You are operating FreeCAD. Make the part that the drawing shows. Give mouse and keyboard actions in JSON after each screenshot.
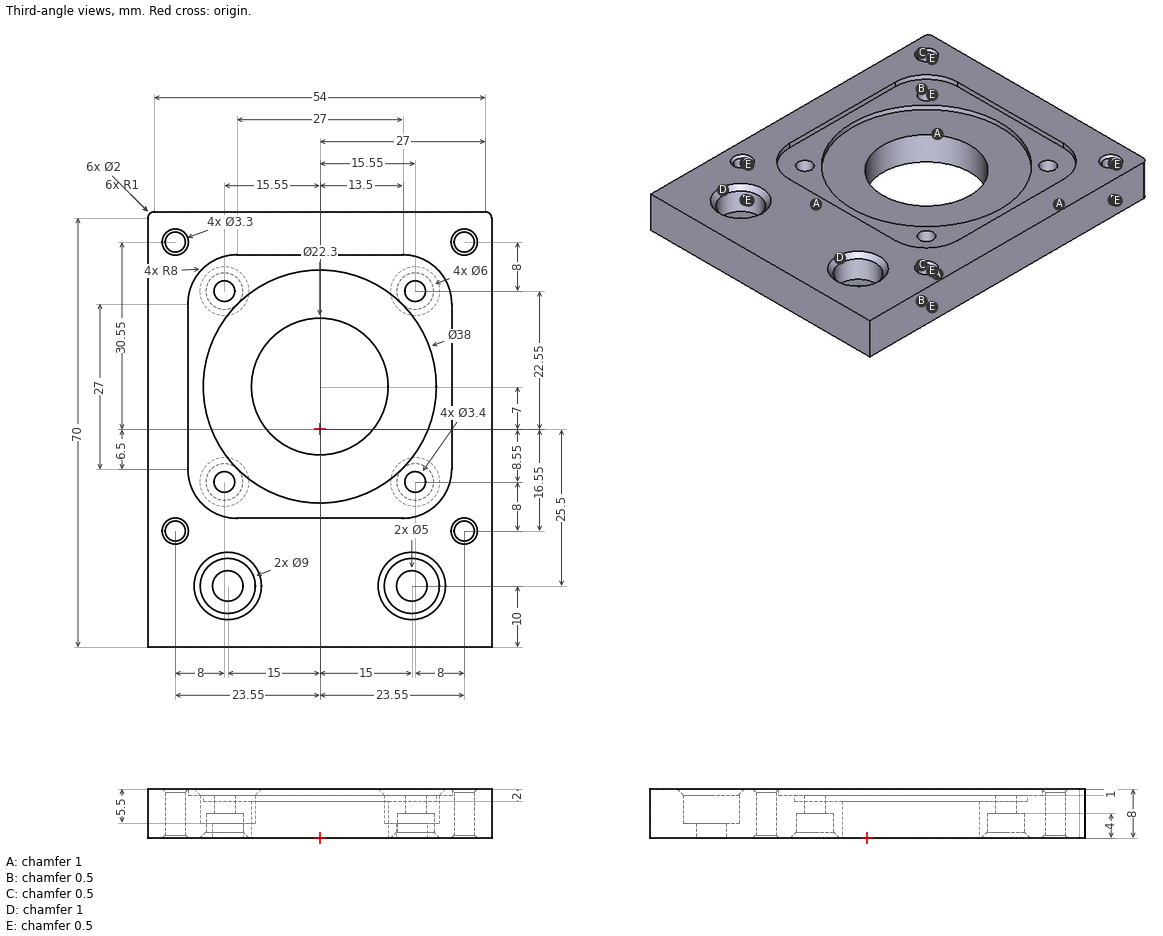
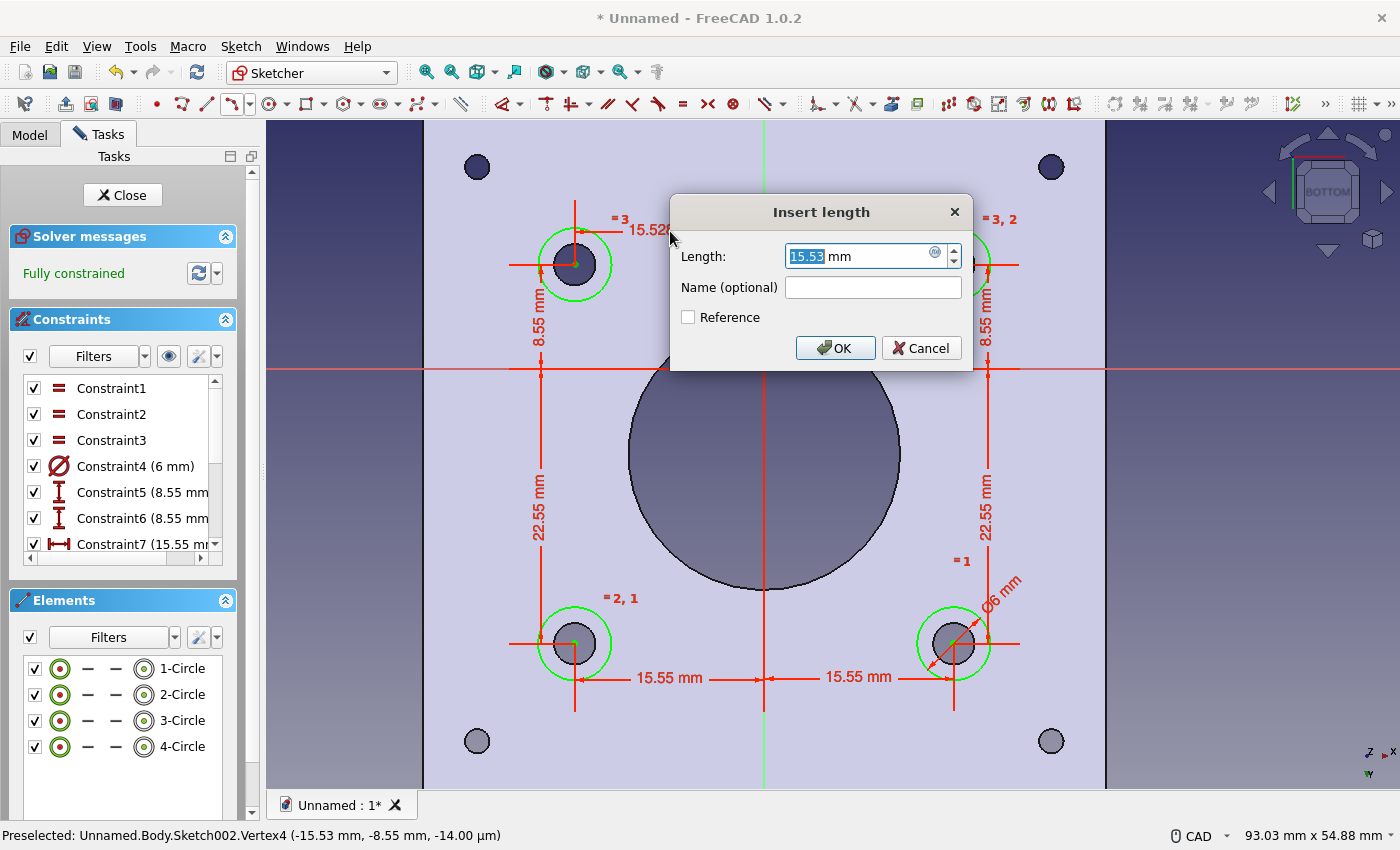
{"action": "type", "text": "15.55"}
{"action": "key", "text": "Return"}
{"action": "key", "text": "Escape"}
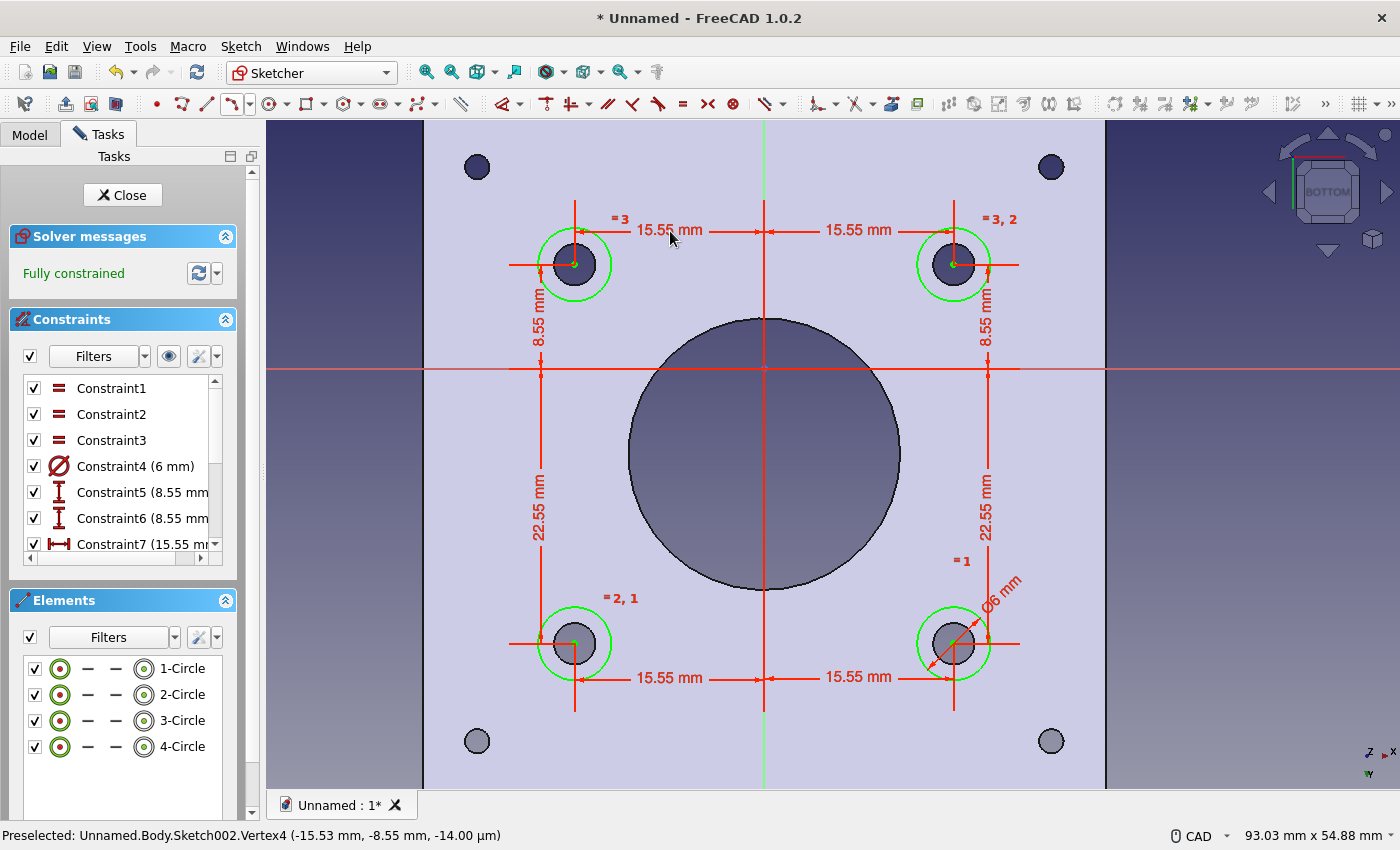
{"action": "left_click", "coordinate": [123, 195]}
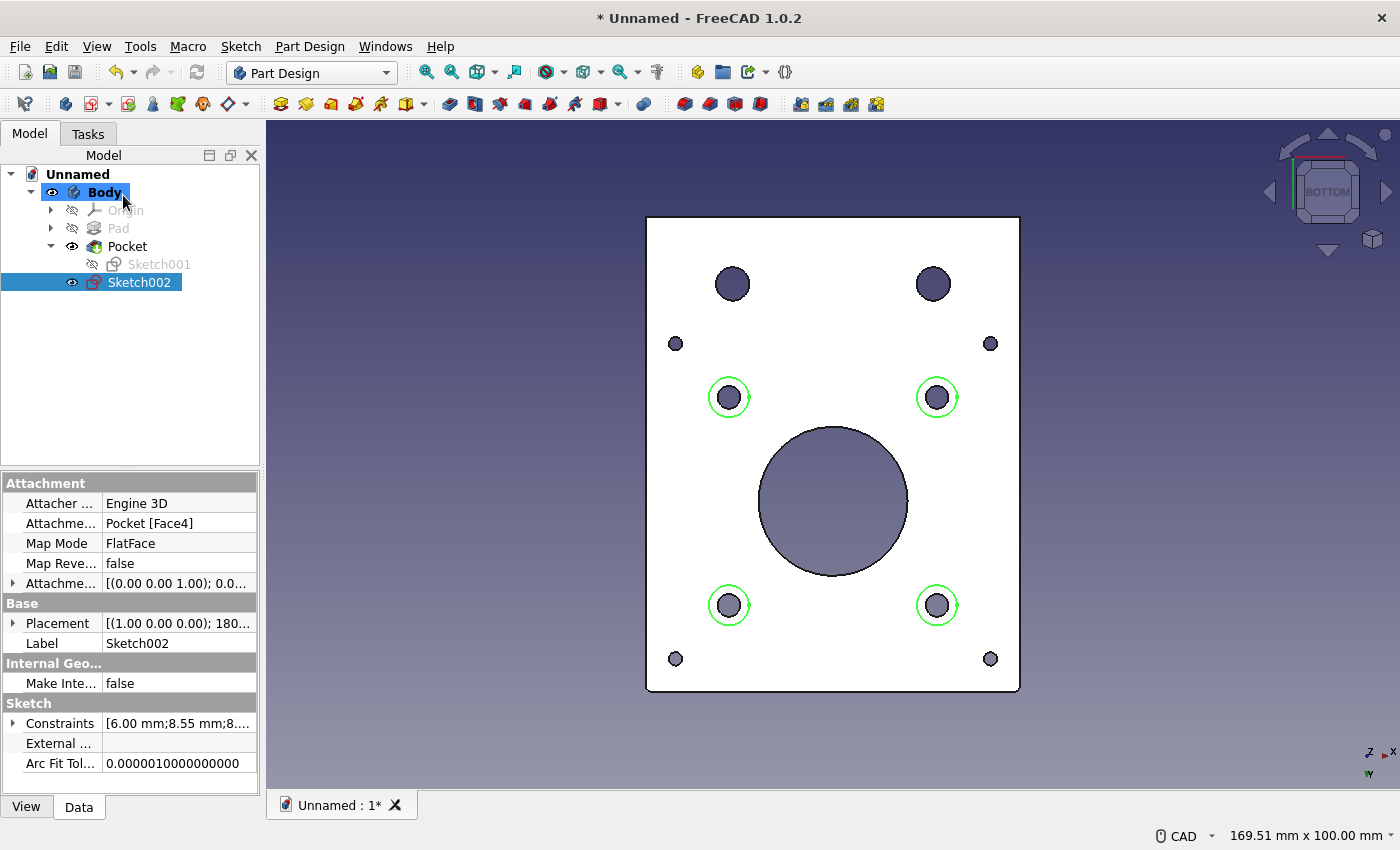
{"action": "left_click", "coordinate": [450, 104]}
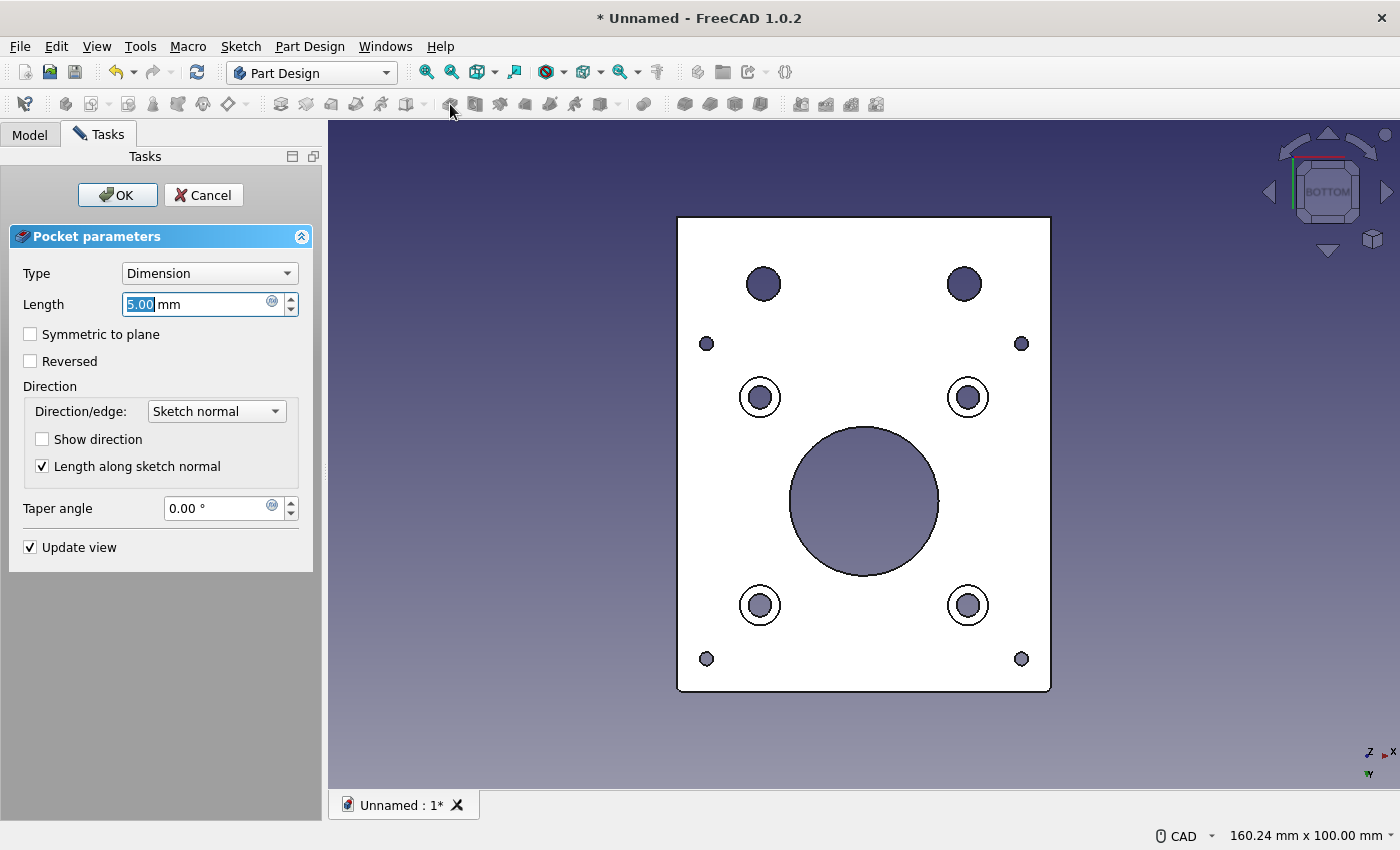
{"action": "type", "text": "4"}
{"action": "key", "text": "Tab"}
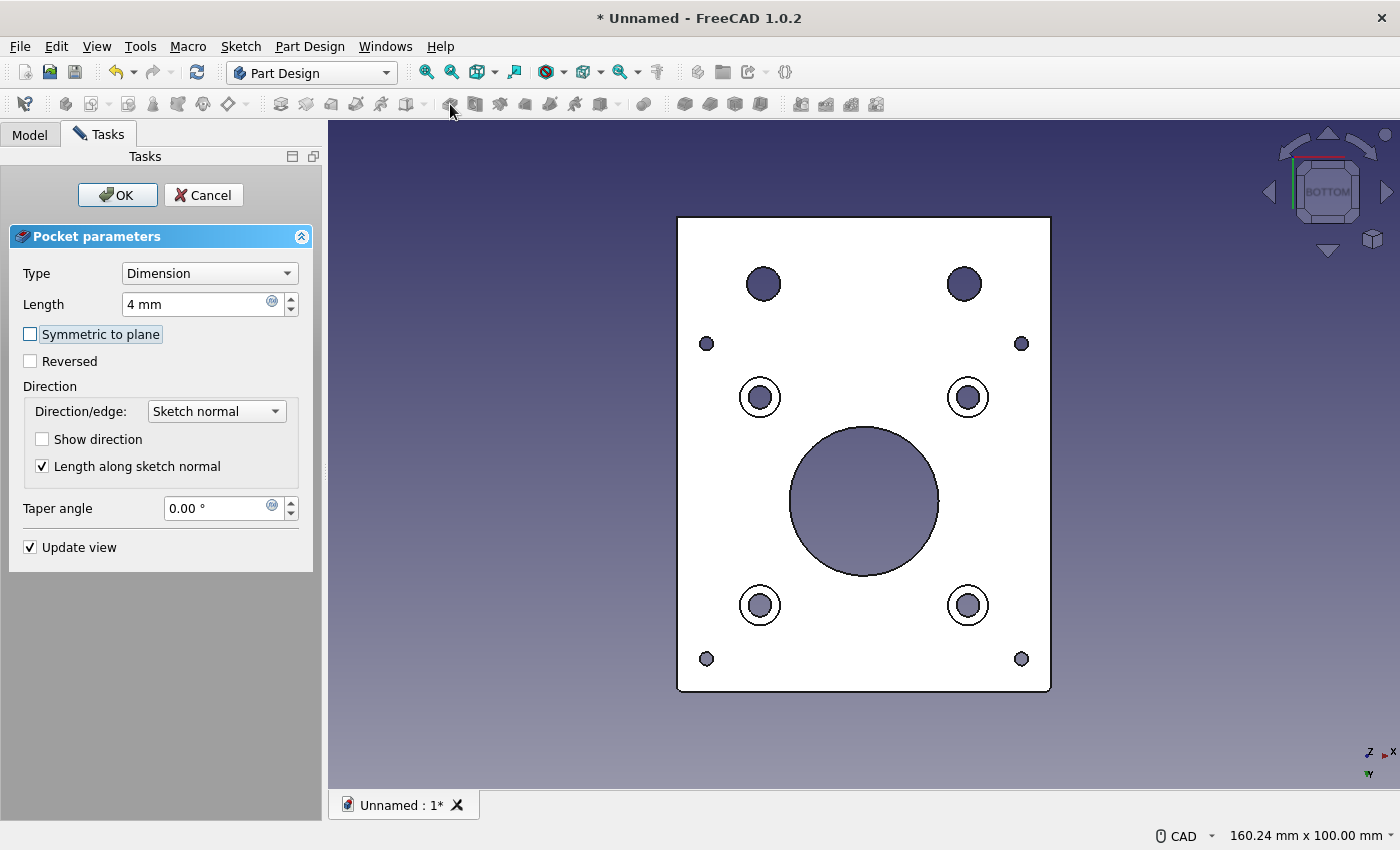
{"action": "left_click", "coordinate": [118, 195]}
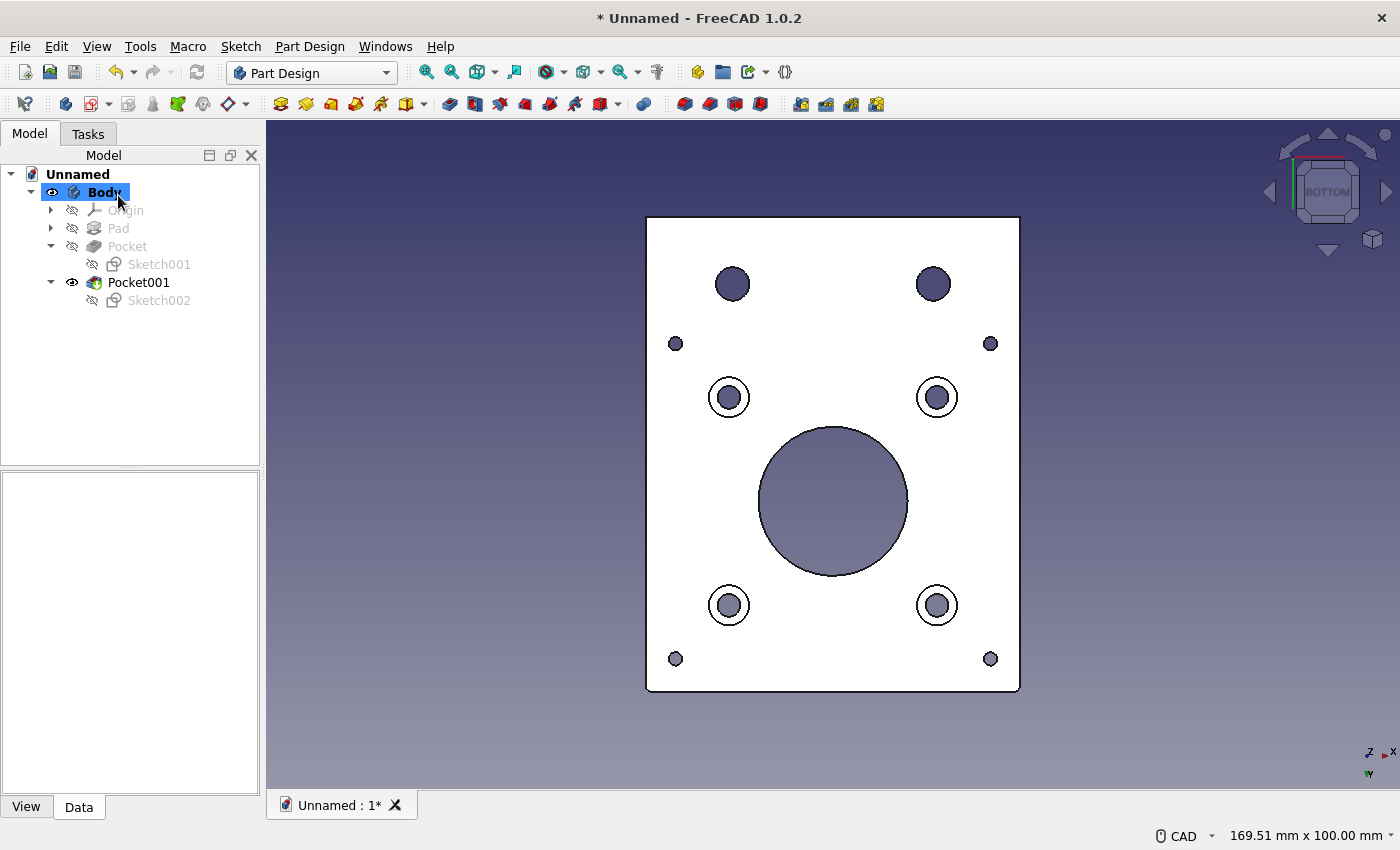
{"action": "left_click", "coordinate": [917, 604]}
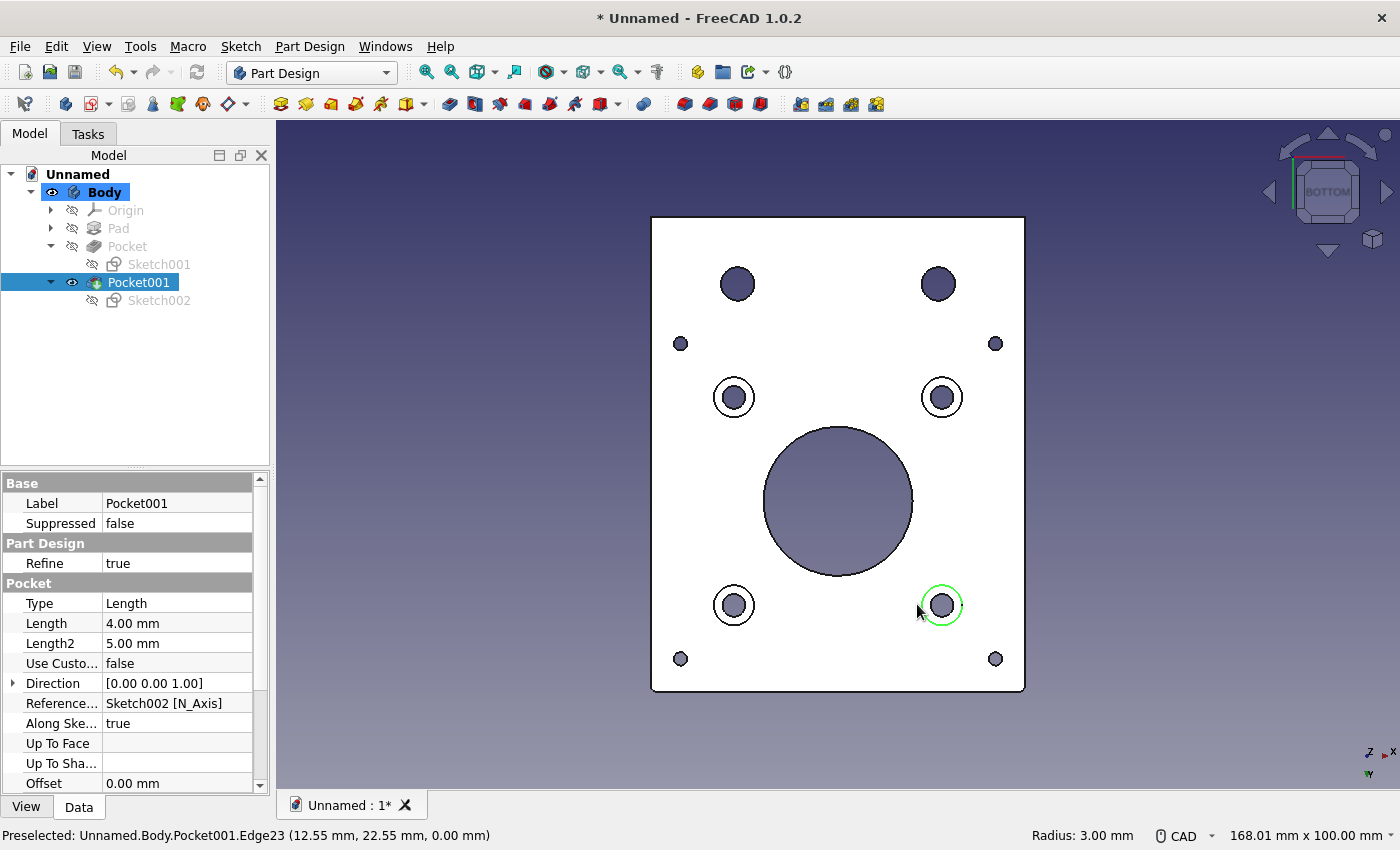
{"action": "left_click", "coordinate": [714, 604], "text": "ctrl"}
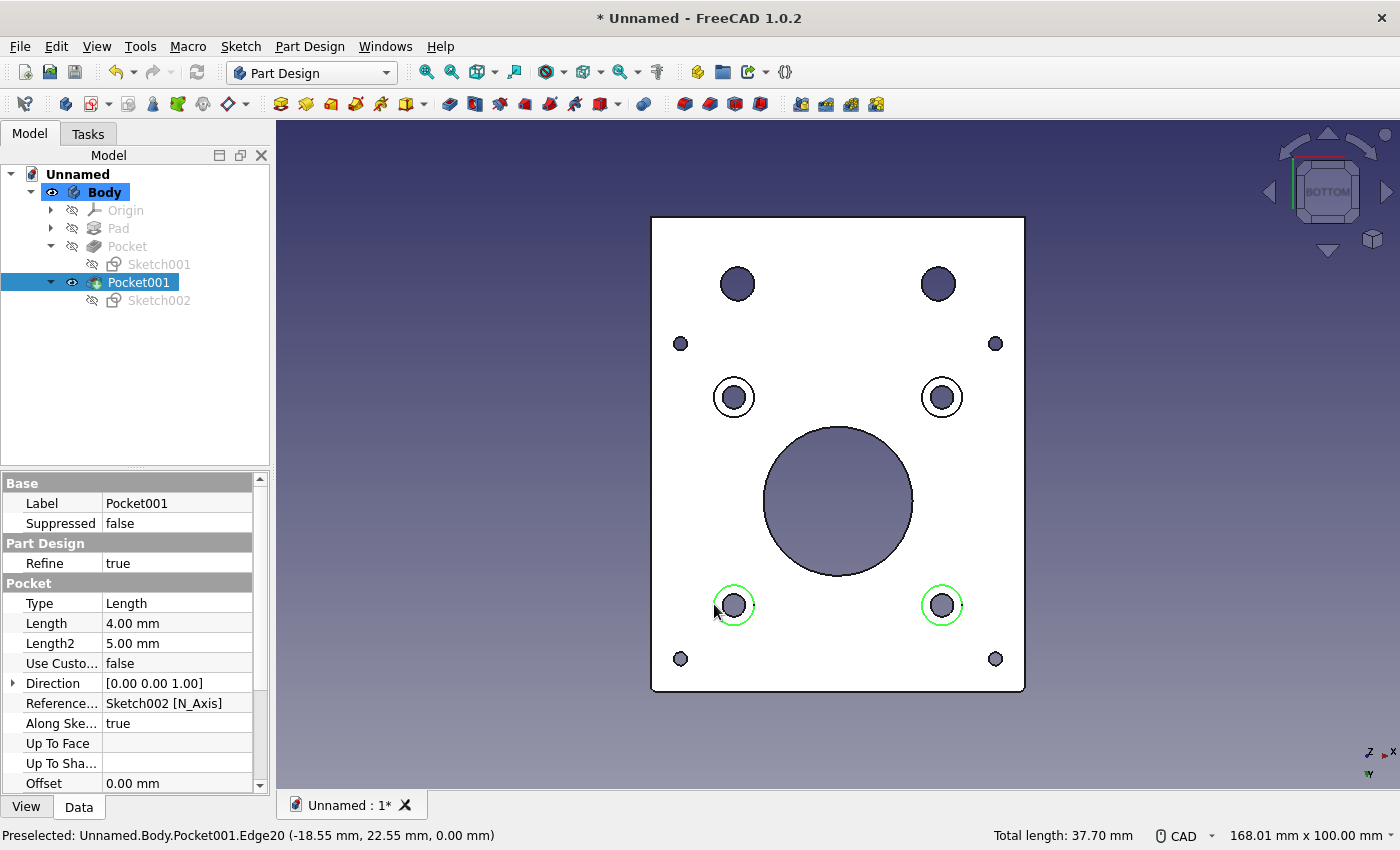
{"action": "left_click", "coordinate": [922, 396], "text": "ctrl"}